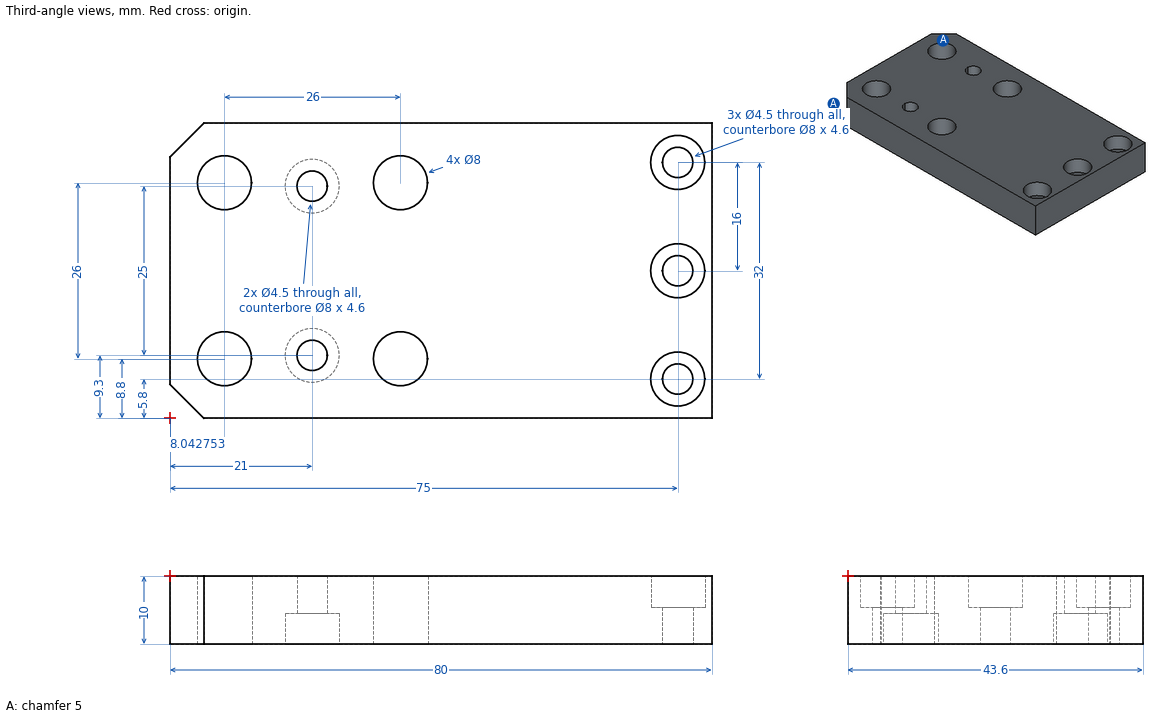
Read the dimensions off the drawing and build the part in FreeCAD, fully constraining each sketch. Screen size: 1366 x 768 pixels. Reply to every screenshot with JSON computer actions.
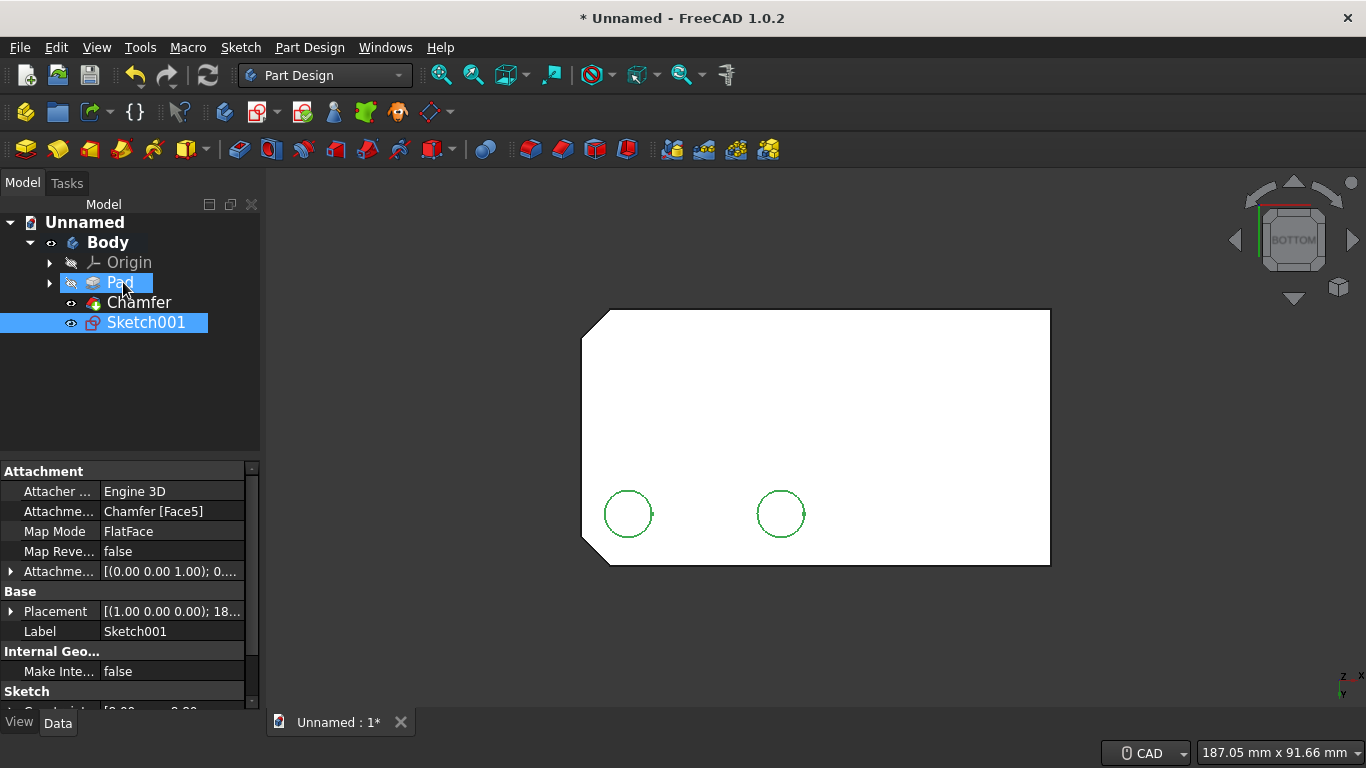
{"action": "left_click", "coordinate": [240, 150]}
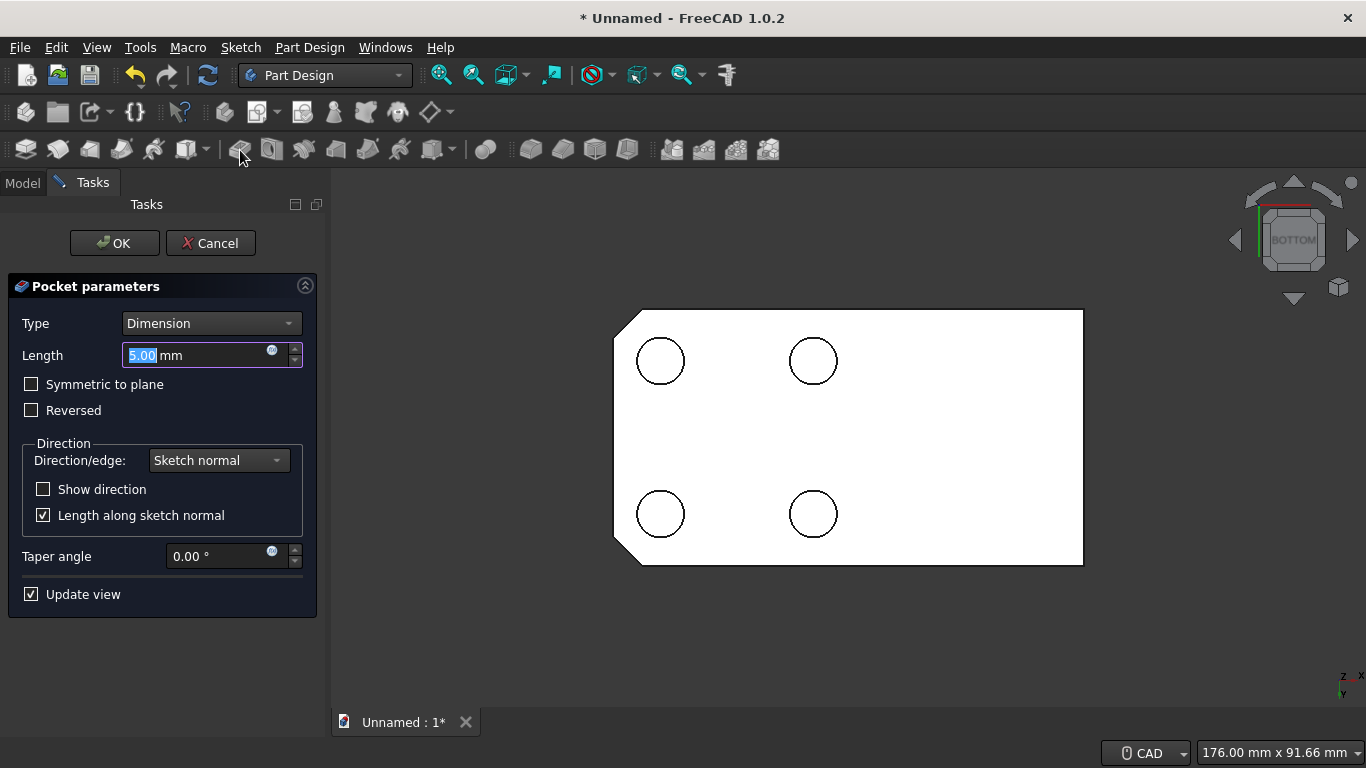
{"action": "left_click", "coordinate": [212, 324]}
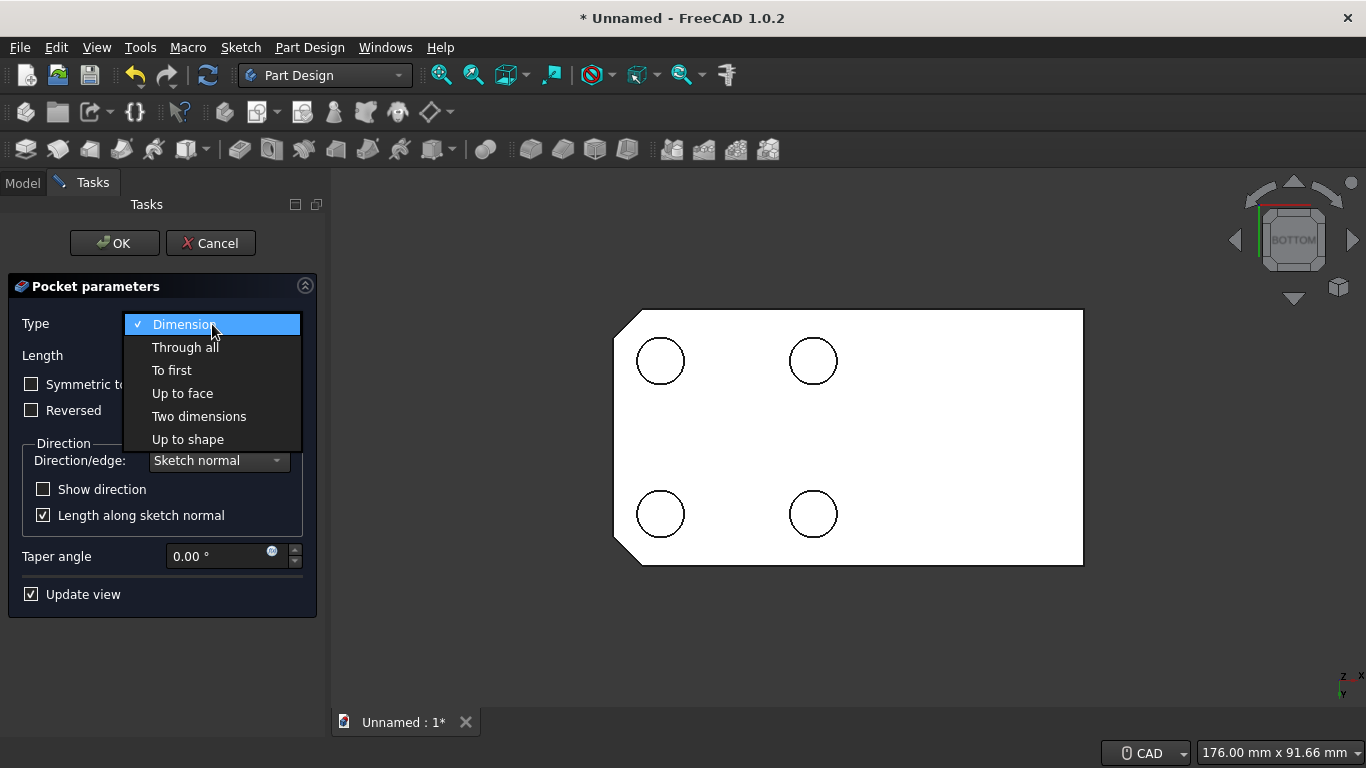
{"action": "left_click", "coordinate": [212, 348]}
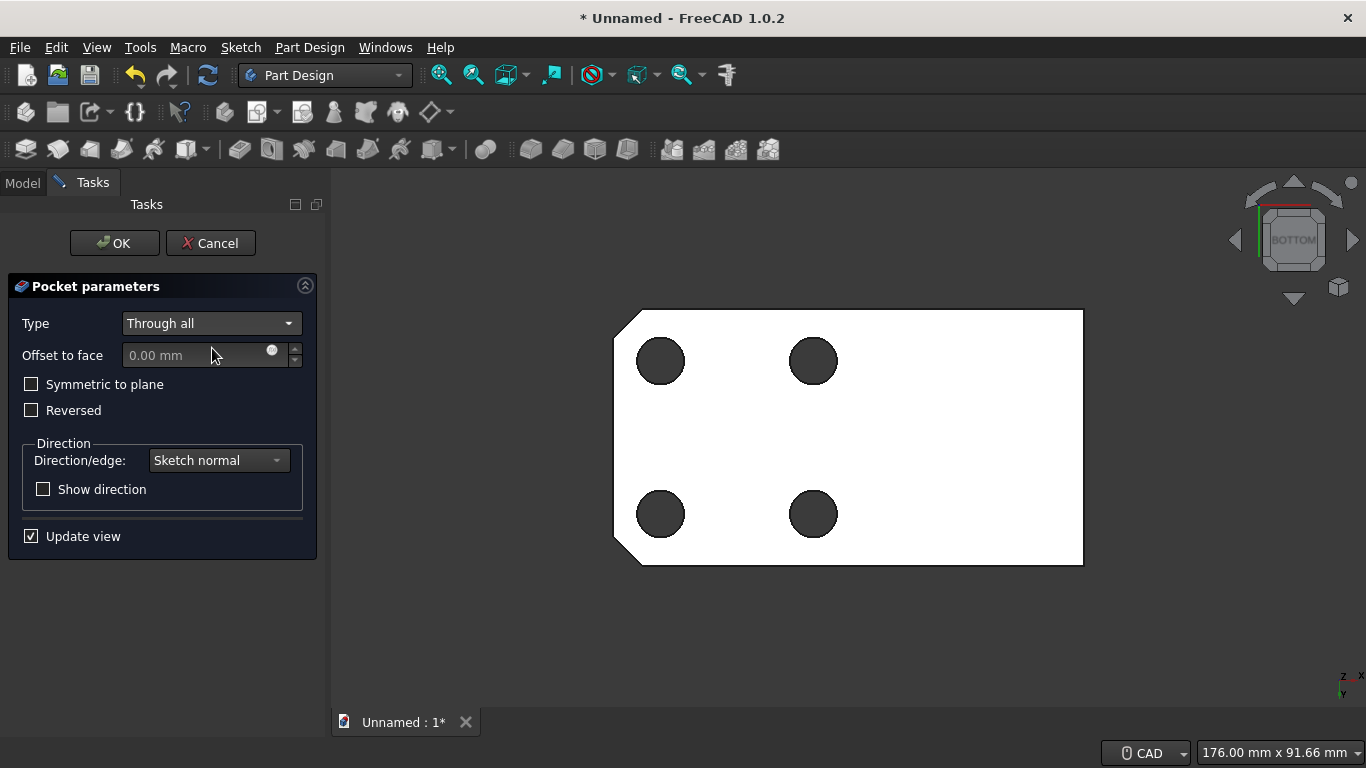
{"action": "left_click", "coordinate": [115, 243]}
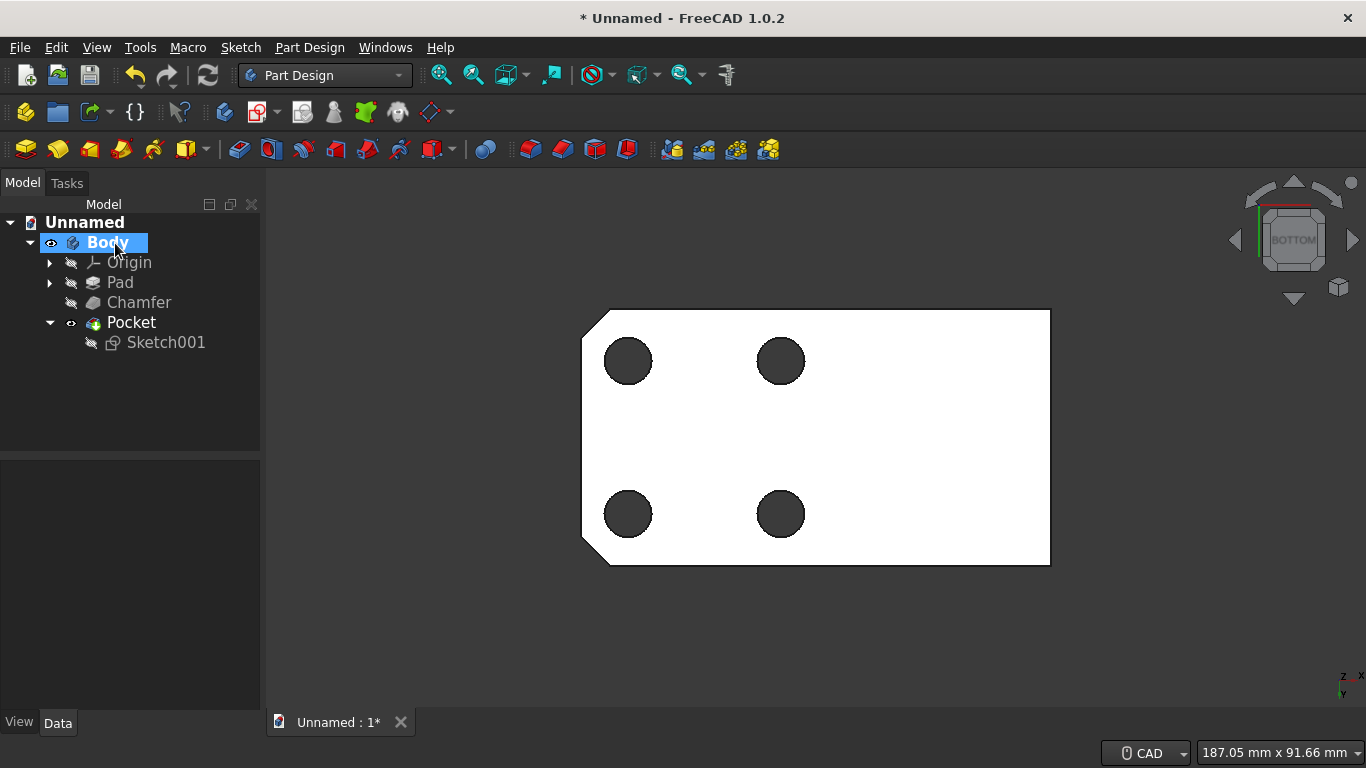
{"action": "left_click", "coordinate": [883, 437]}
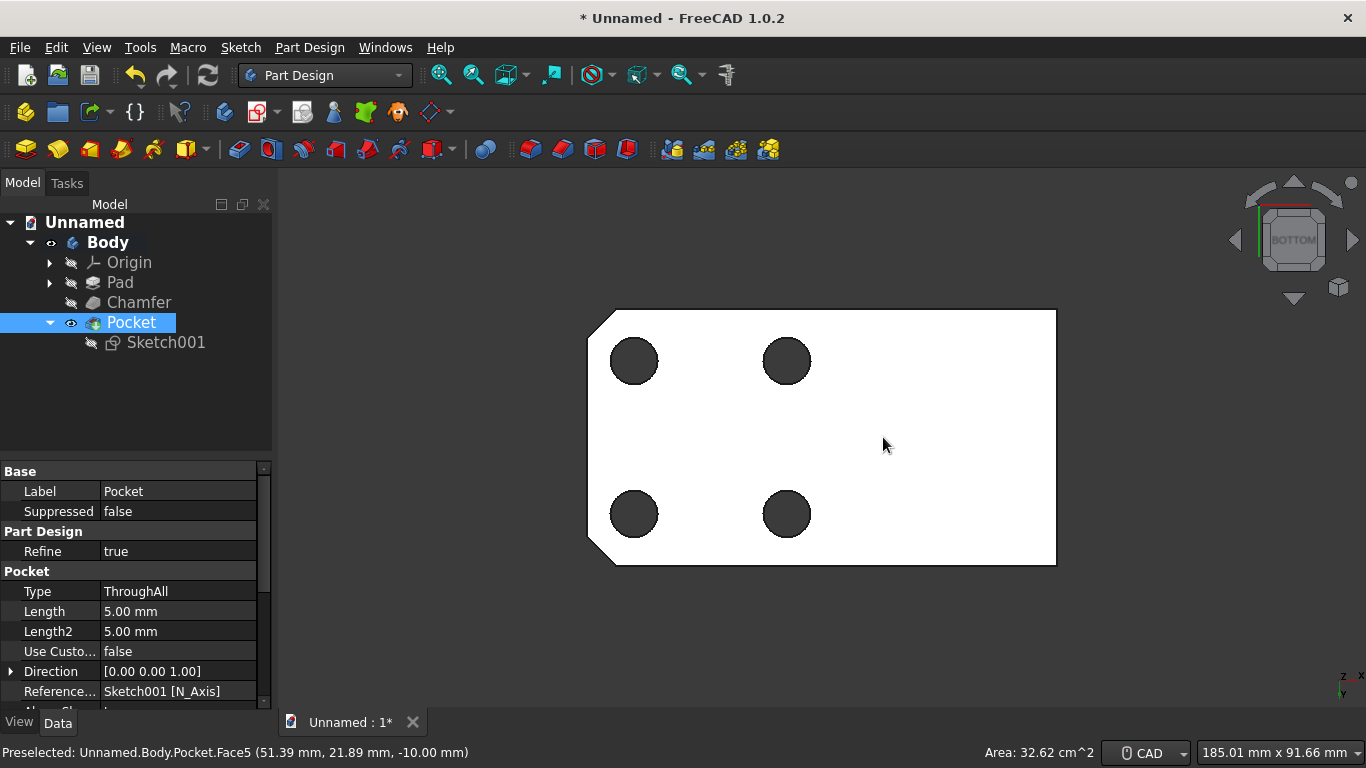
{"action": "left_click", "coordinate": [258, 112]}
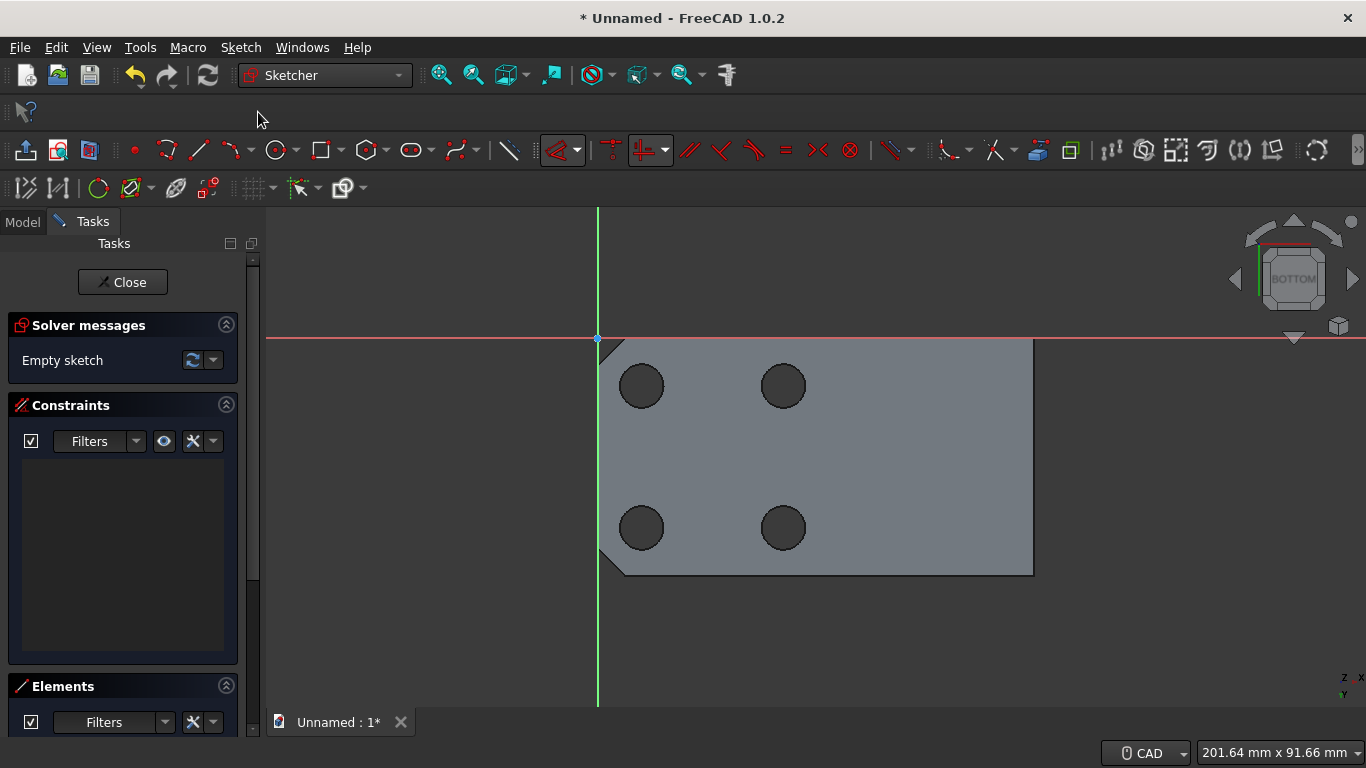
{"action": "scroll", "coordinate": [486, 399], "scroll_direction": "up", "scroll_amount": 2}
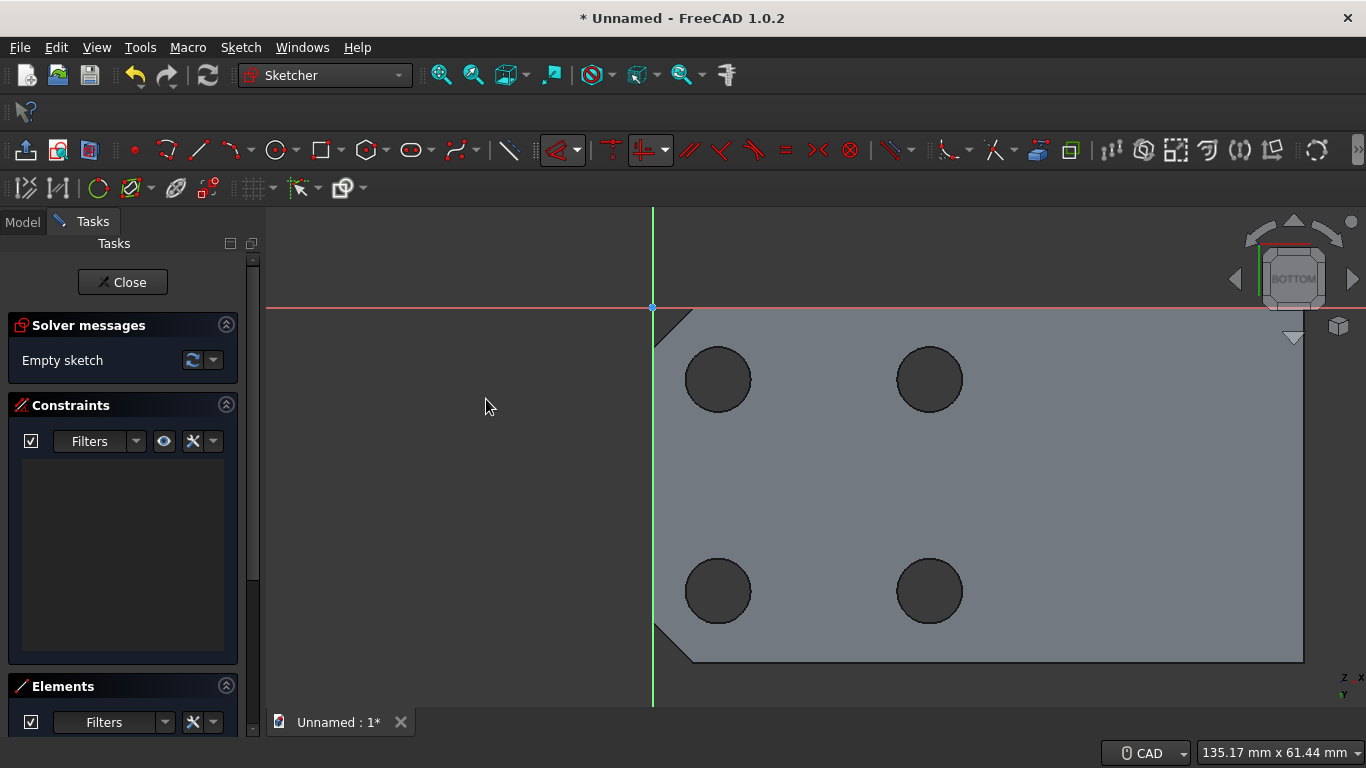
{"action": "left_click", "coordinate": [276, 150]}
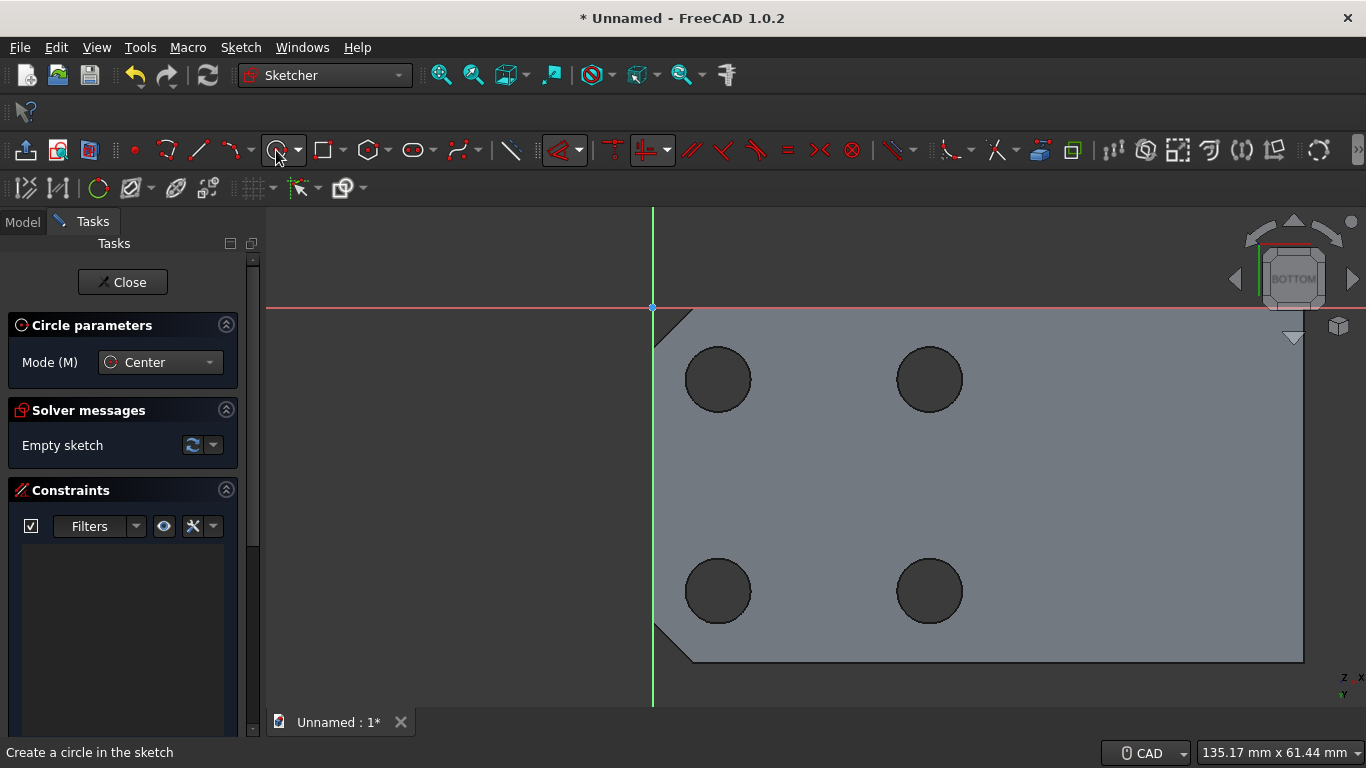
{"action": "scroll", "coordinate": [824, 587], "scroll_direction": "up", "scroll_amount": 2}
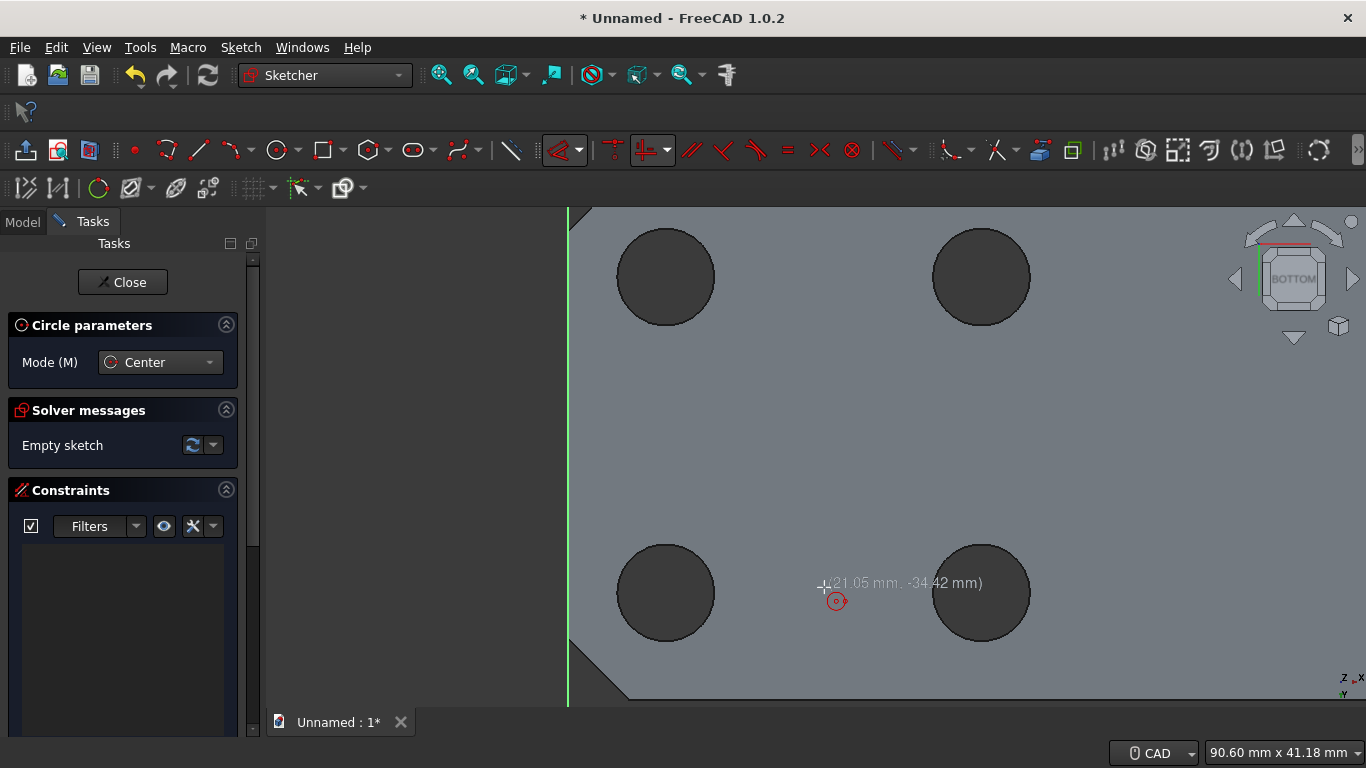
{"action": "left_click", "coordinate": [823, 587]}
{"action": "left_click", "coordinate": [842, 567]}